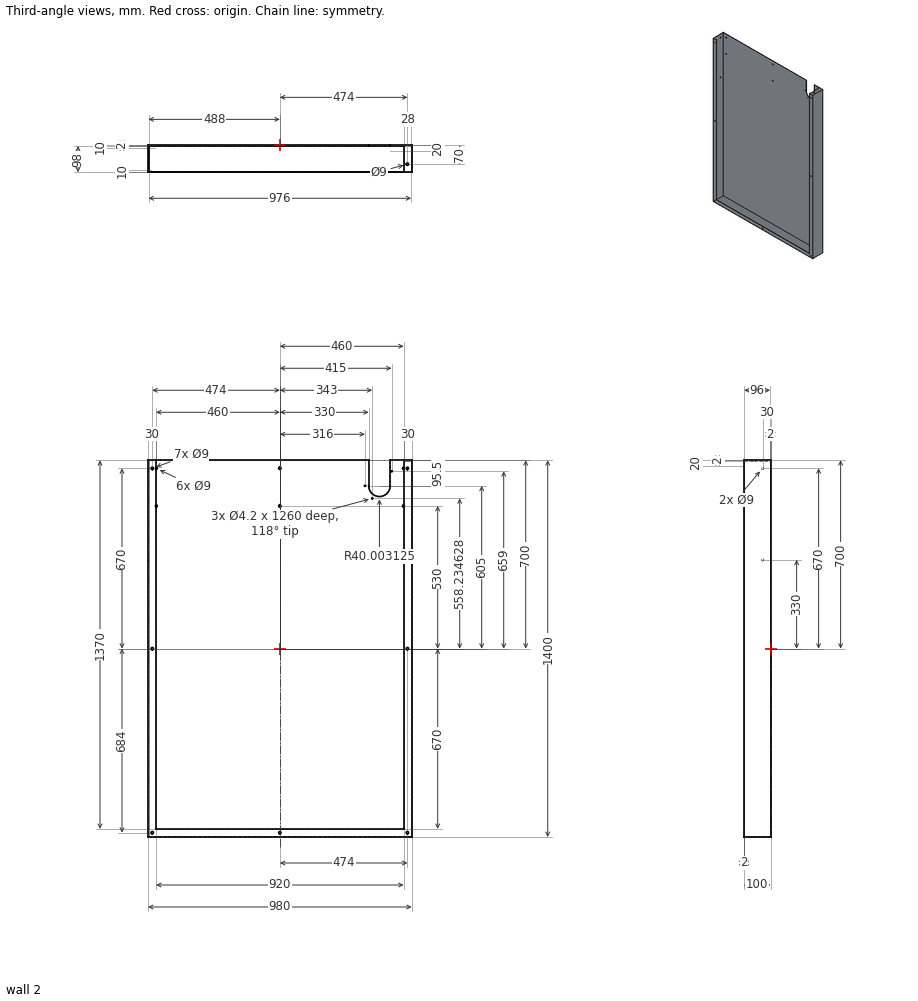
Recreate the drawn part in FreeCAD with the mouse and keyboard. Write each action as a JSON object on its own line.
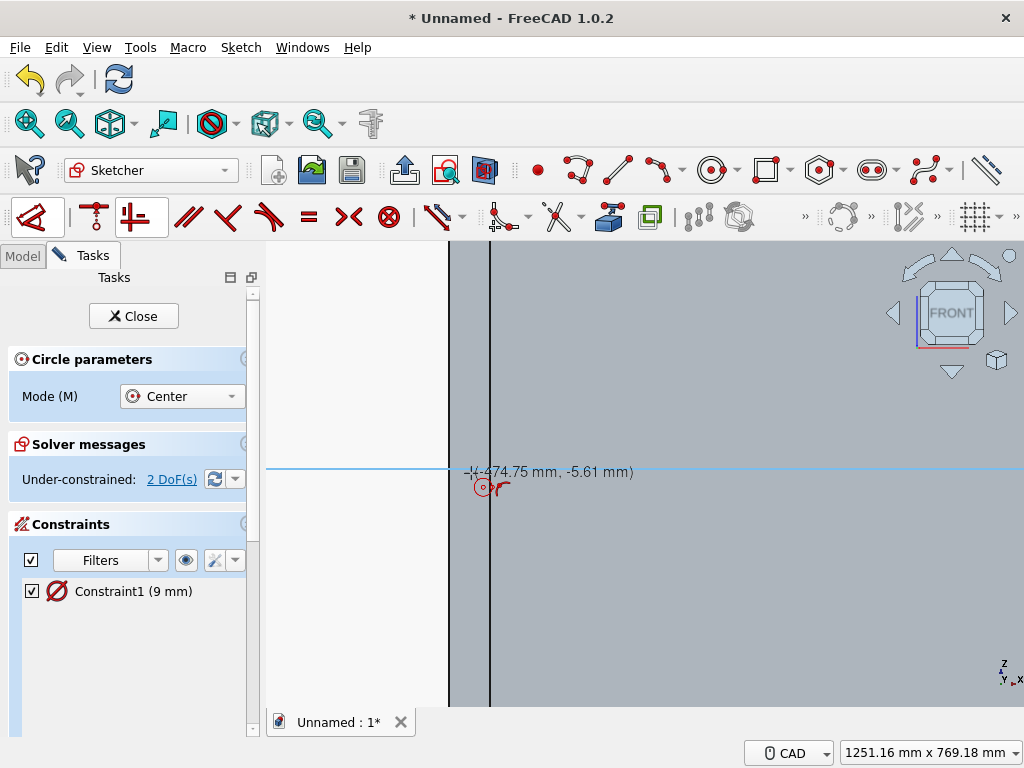
{"action": "scroll", "coordinate": [471, 473], "scroll_direction": "down", "scroll_amount": 16}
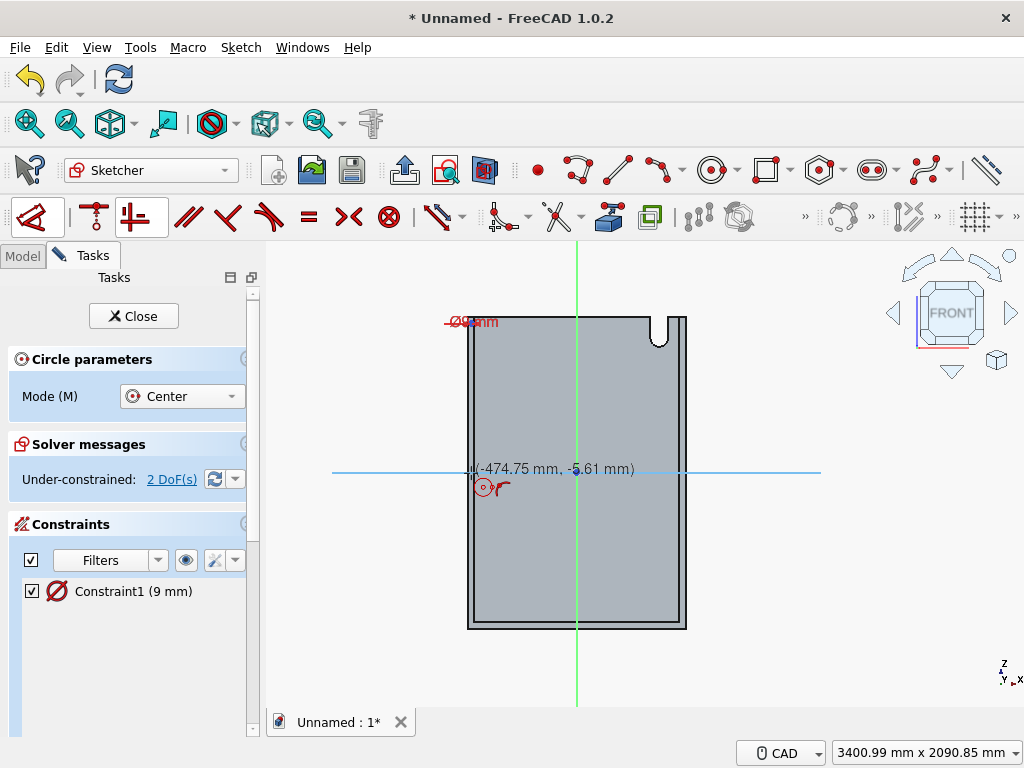
{"action": "left_click", "coordinate": [471, 473]}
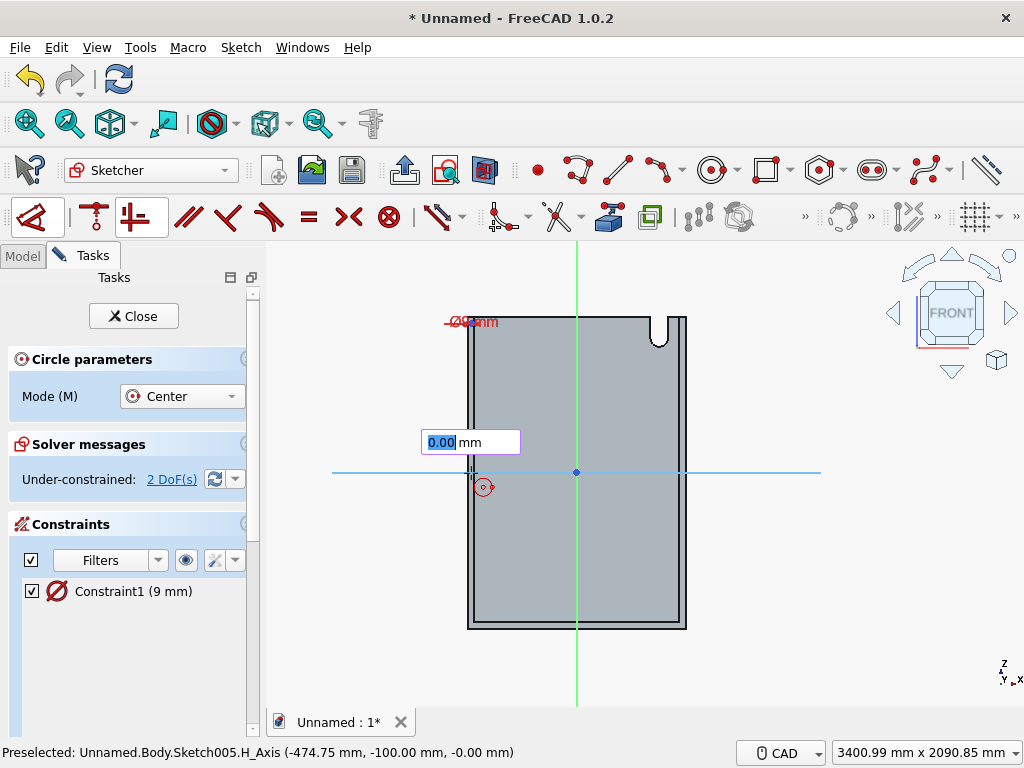
{"action": "scroll", "coordinate": [471, 474], "scroll_direction": "up", "scroll_amount": 15}
{"action": "mouse_move", "coordinate": [462, 458]}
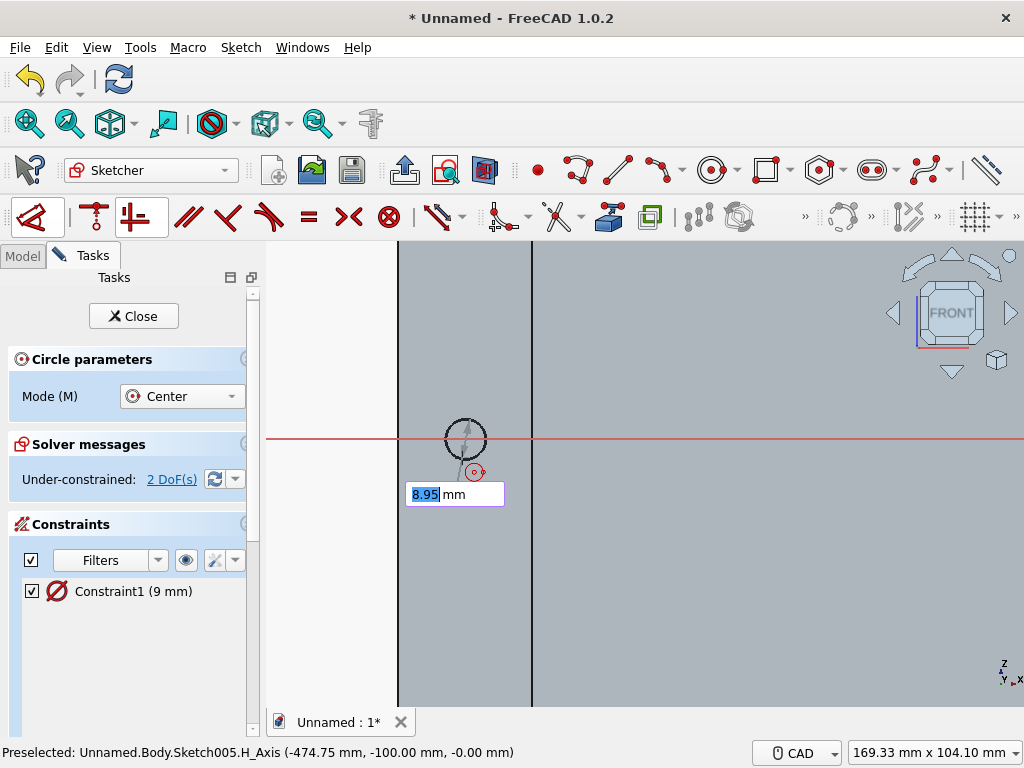
{"action": "type", "text": "9"}
{"action": "key", "text": "Return"}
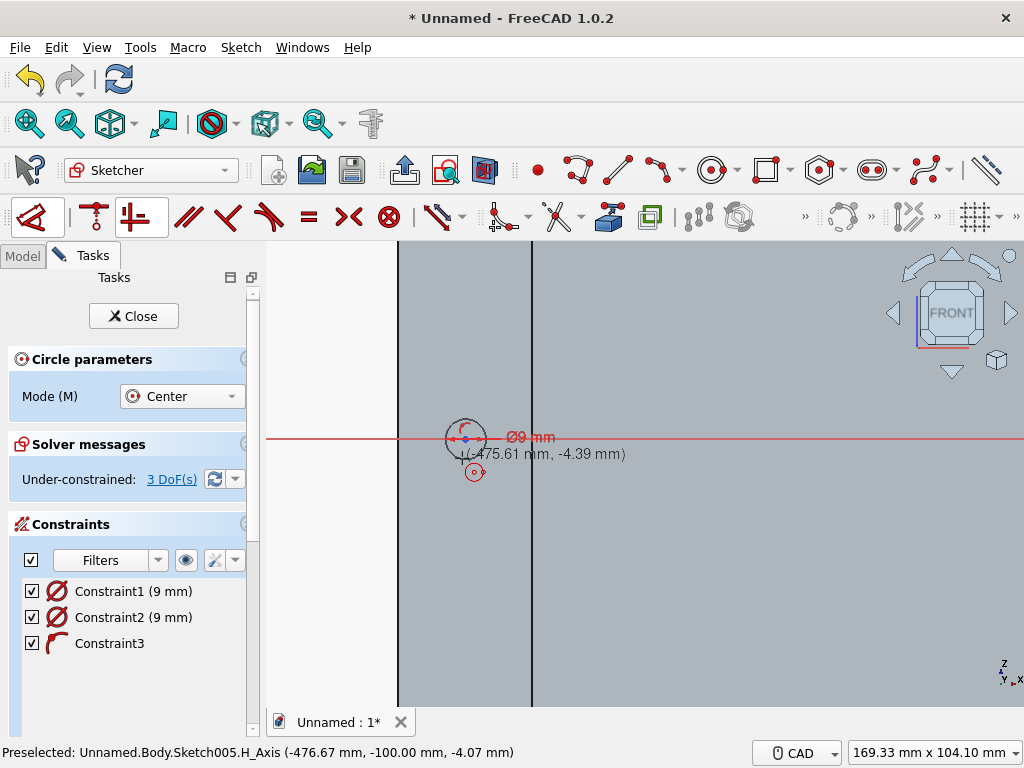
{"action": "scroll", "coordinate": [471, 474], "scroll_direction": "down", "scroll_amount": 15}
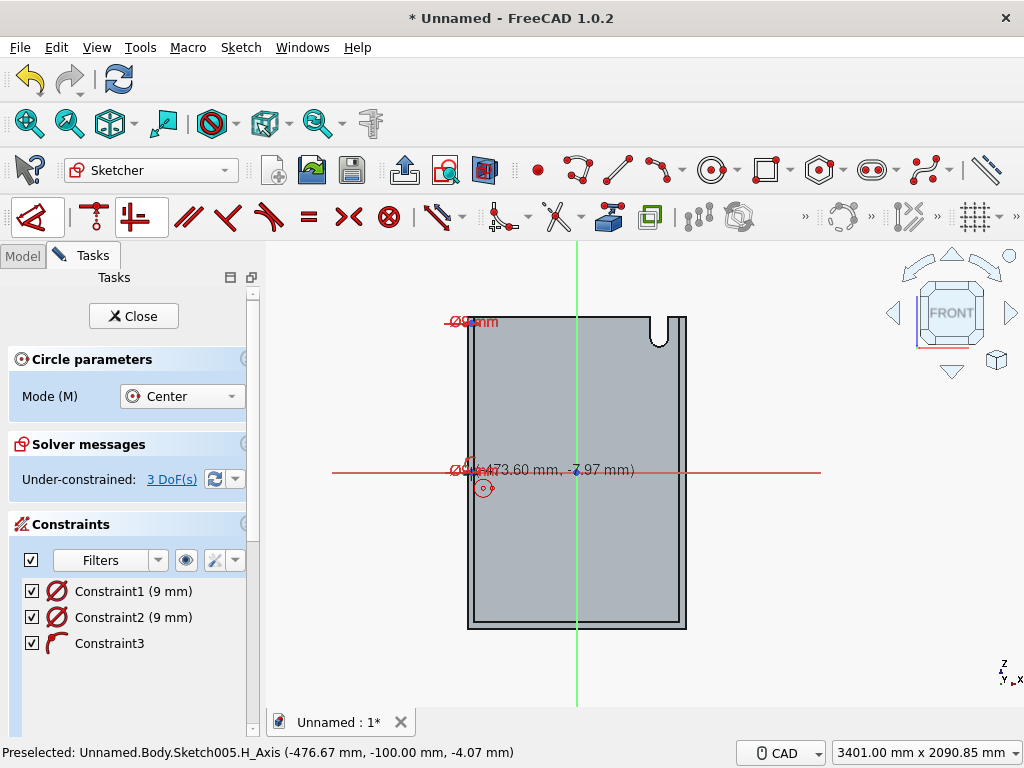
{"action": "scroll", "coordinate": [471, 625], "scroll_direction": "up", "scroll_amount": 16}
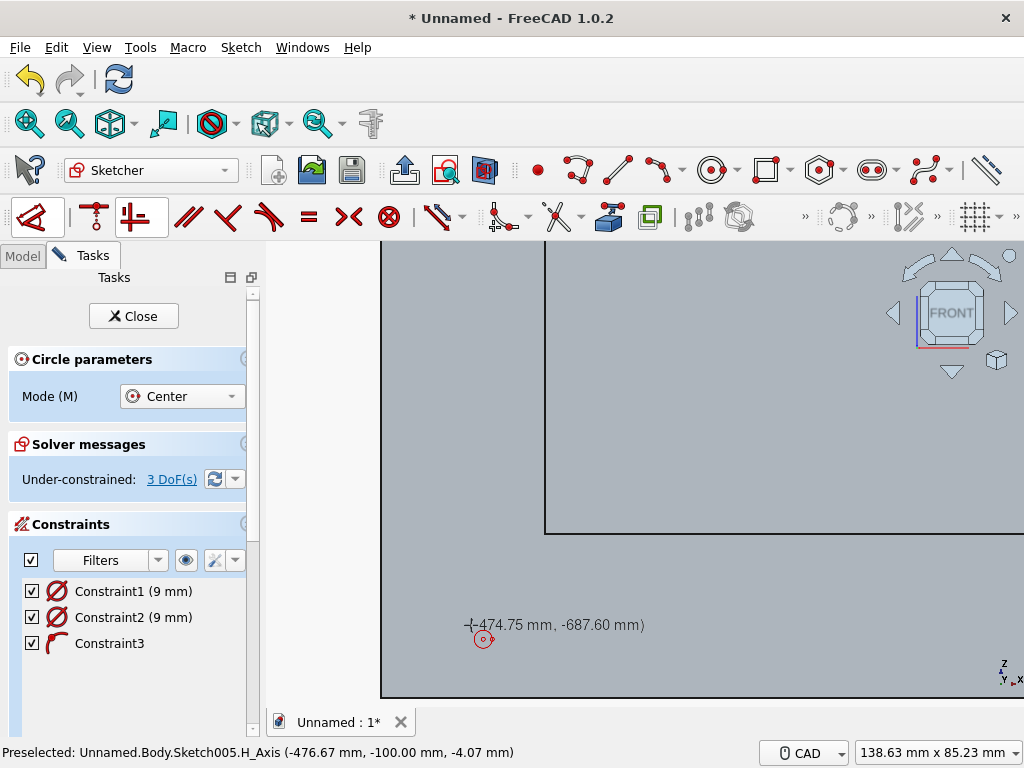
{"action": "scroll", "coordinate": [471, 626], "scroll_direction": "down", "scroll_amount": 16}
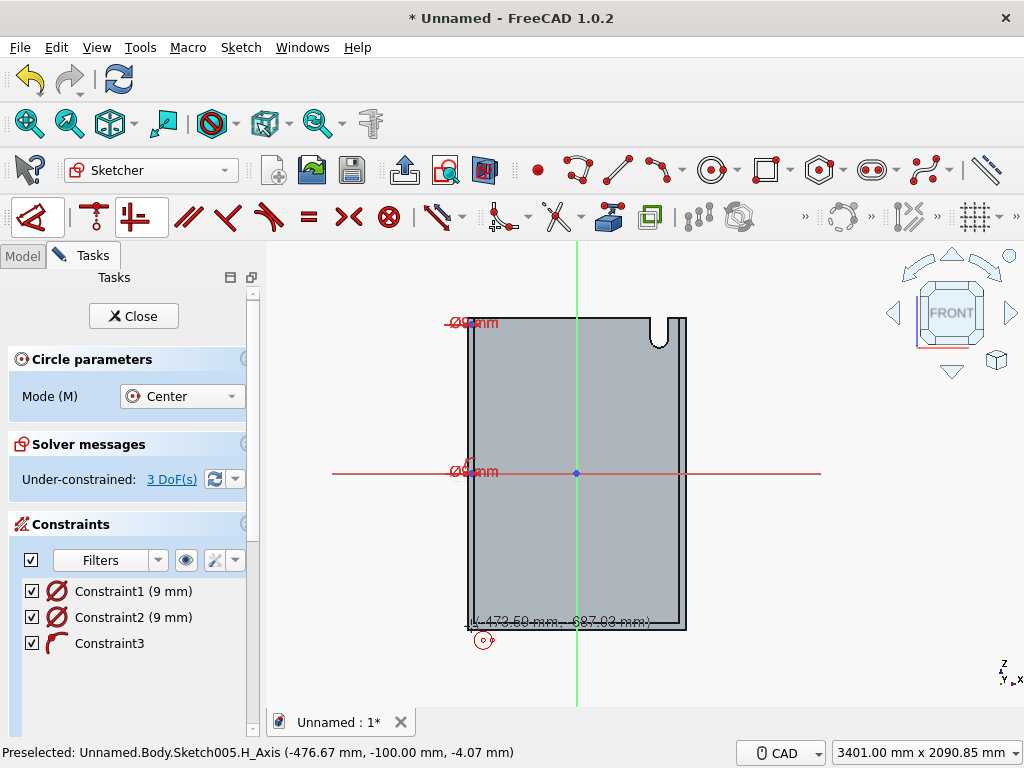
{"action": "left_click", "coordinate": [471, 626]}
{"action": "mouse_move", "coordinate": [472, 625]}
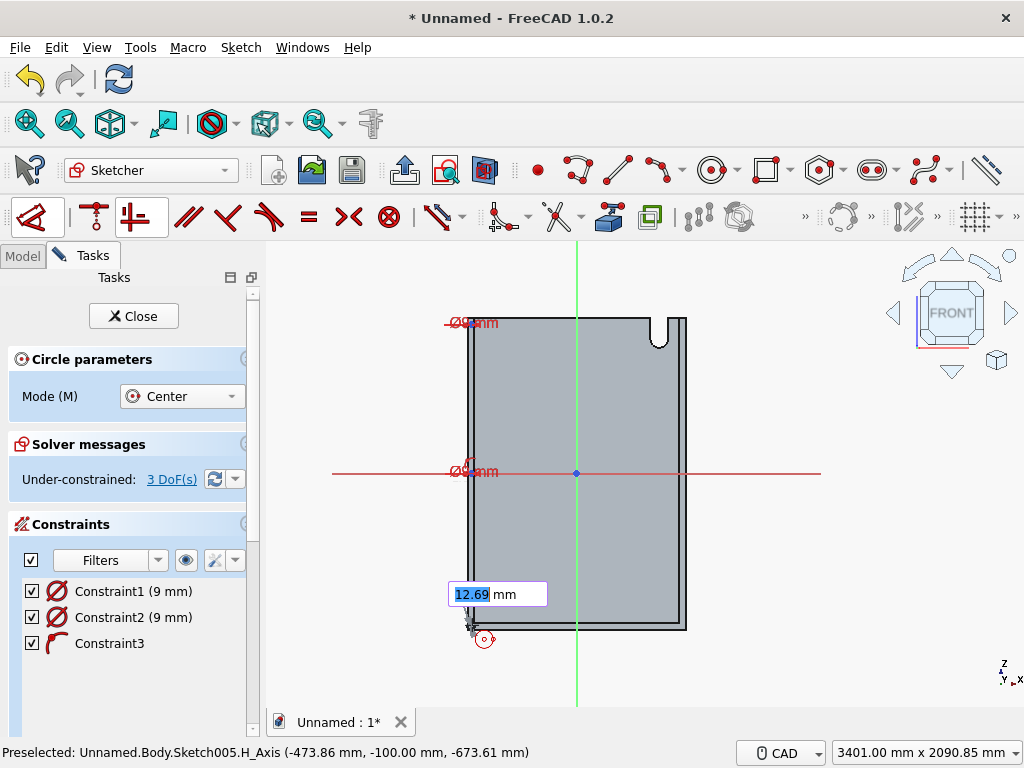
{"action": "type", "text": "9"}
{"action": "key", "text": "Return"}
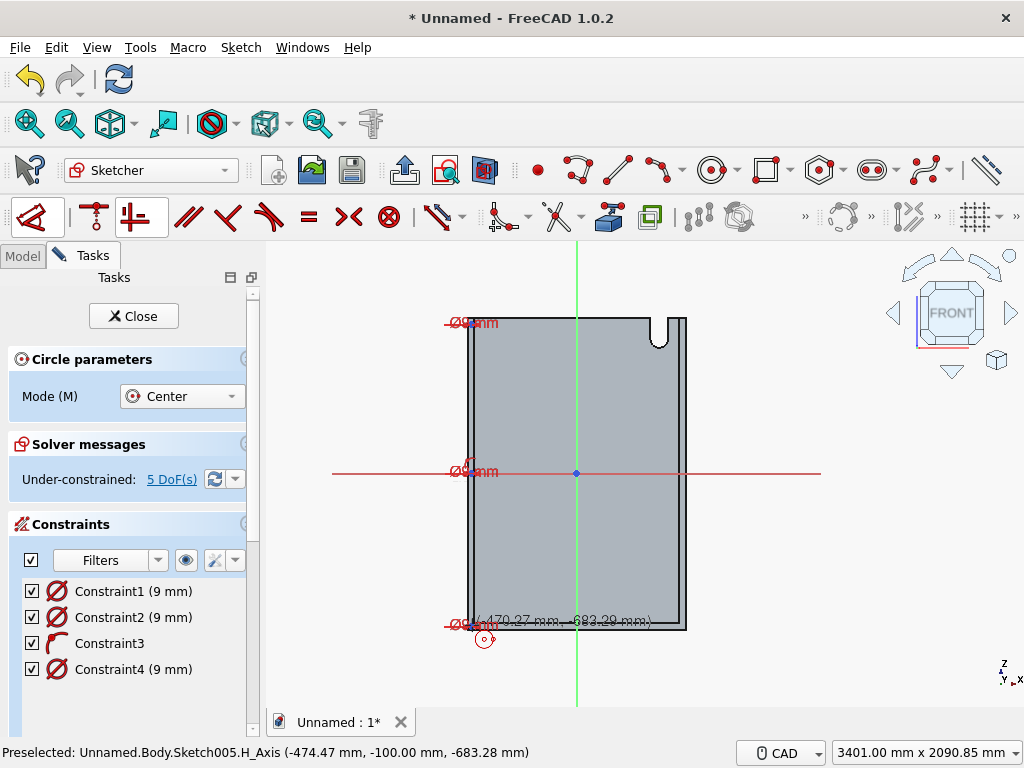
{"action": "scroll", "coordinate": [577, 626], "scroll_direction": "up", "scroll_amount": 16}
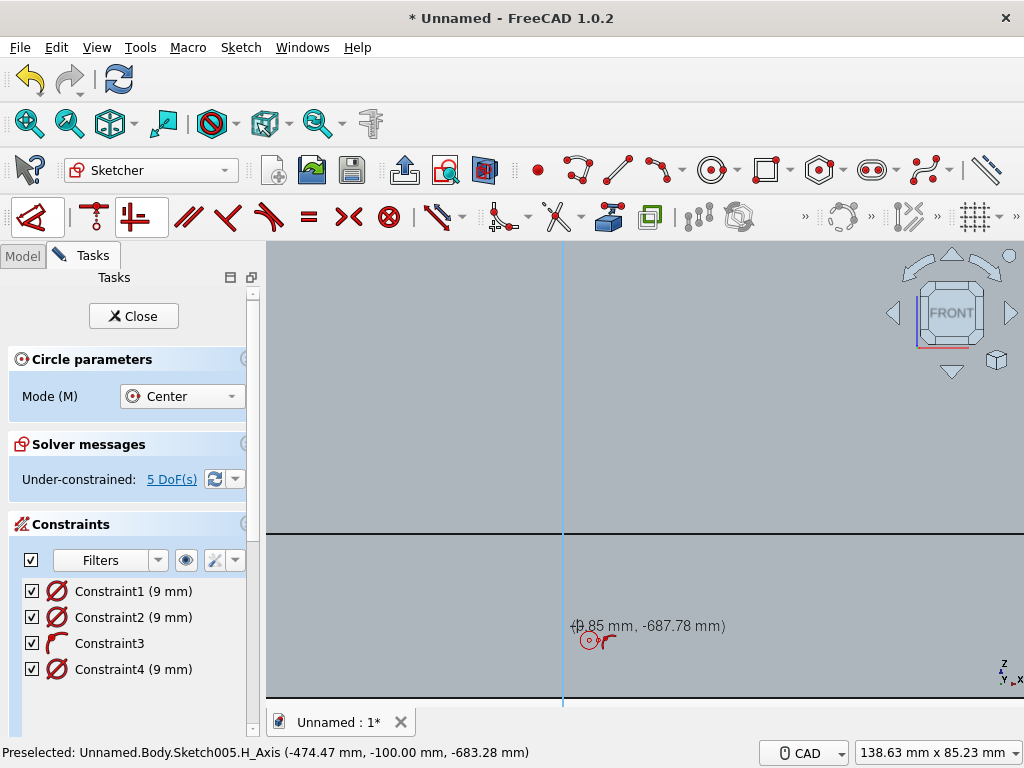
{"action": "scroll", "coordinate": [577, 626], "scroll_direction": "down", "scroll_amount": 16}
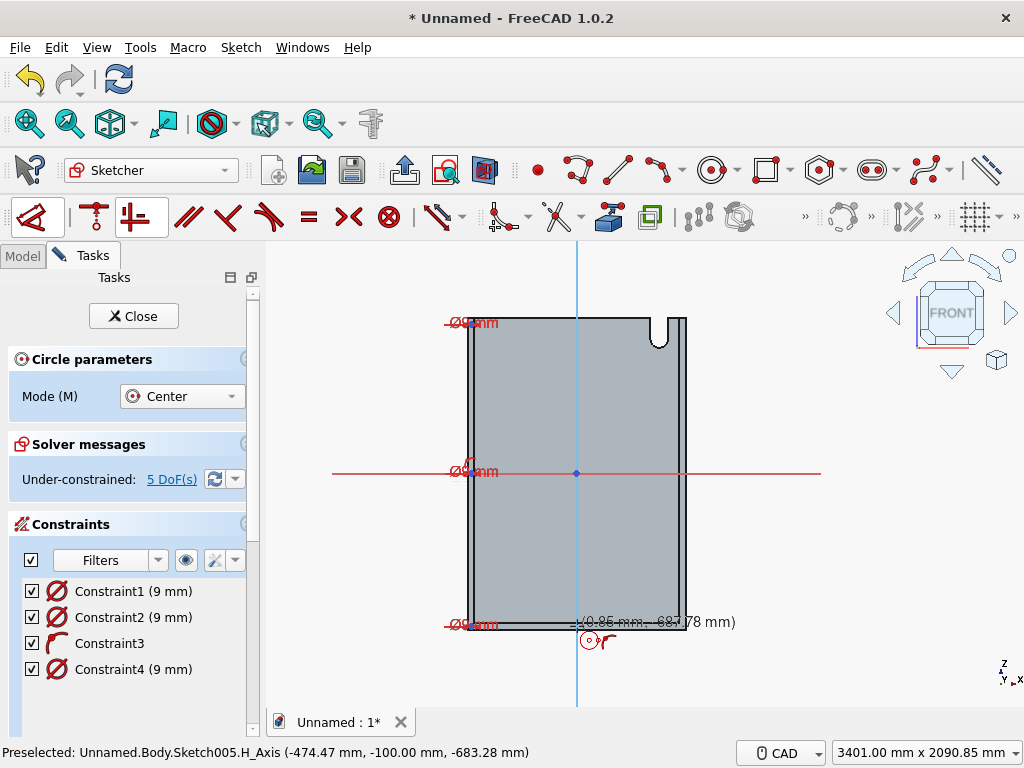
{"action": "left_click", "coordinate": [577, 626]}